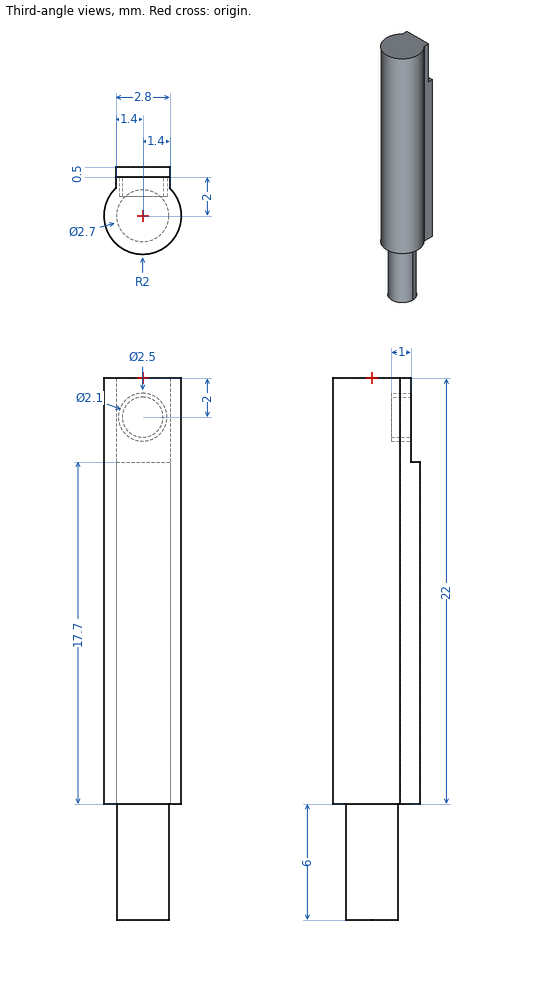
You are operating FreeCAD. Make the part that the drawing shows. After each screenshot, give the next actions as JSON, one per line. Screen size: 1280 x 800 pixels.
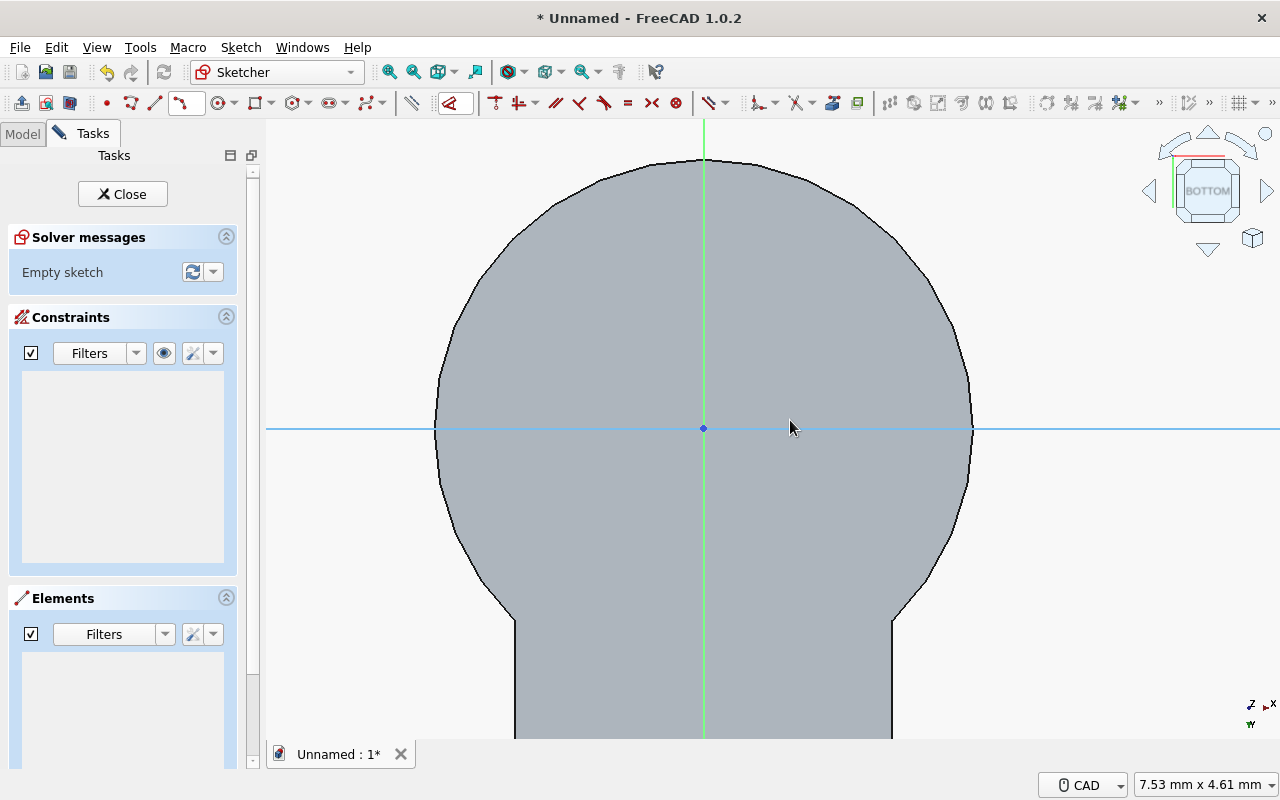
{"action": "left_click", "coordinate": [218, 104]}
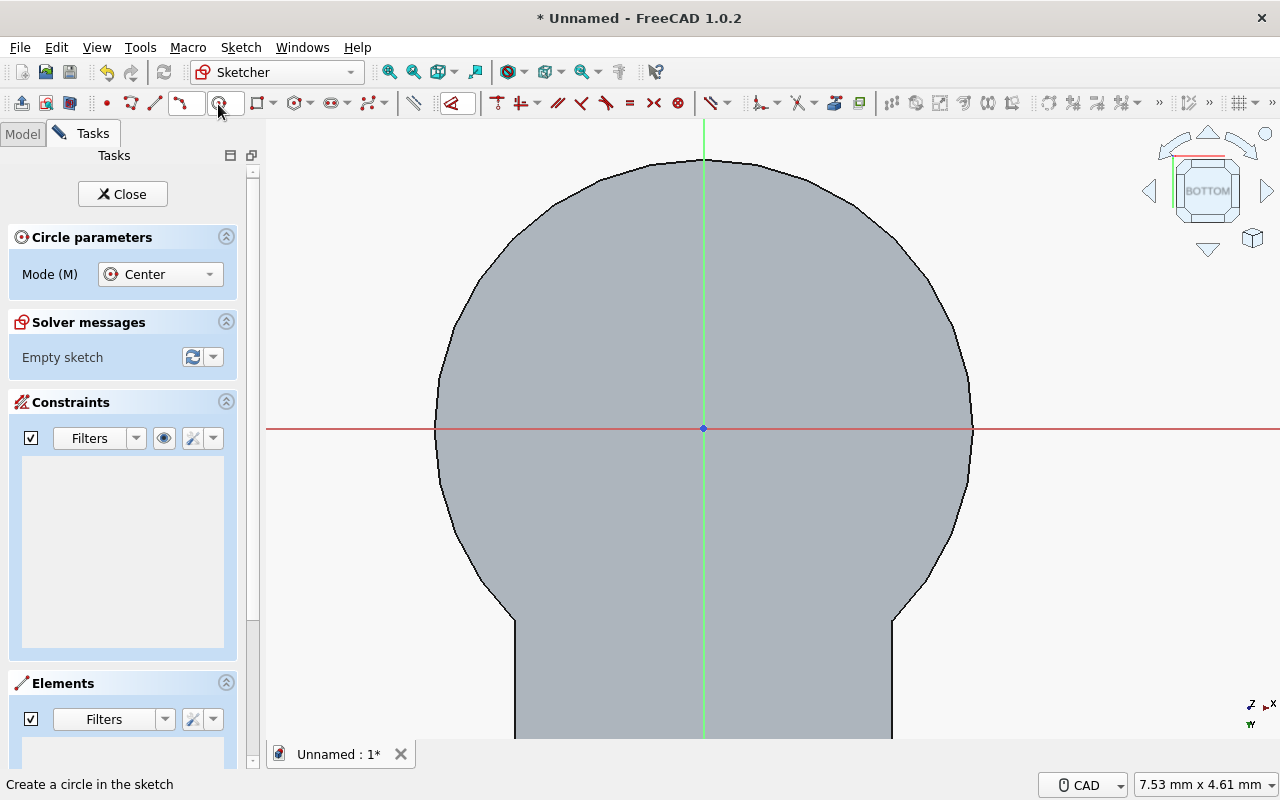
{"action": "left_click", "coordinate": [704, 429]}
{"action": "left_click", "coordinate": [832, 300]}
{"action": "key", "text": "Escape"}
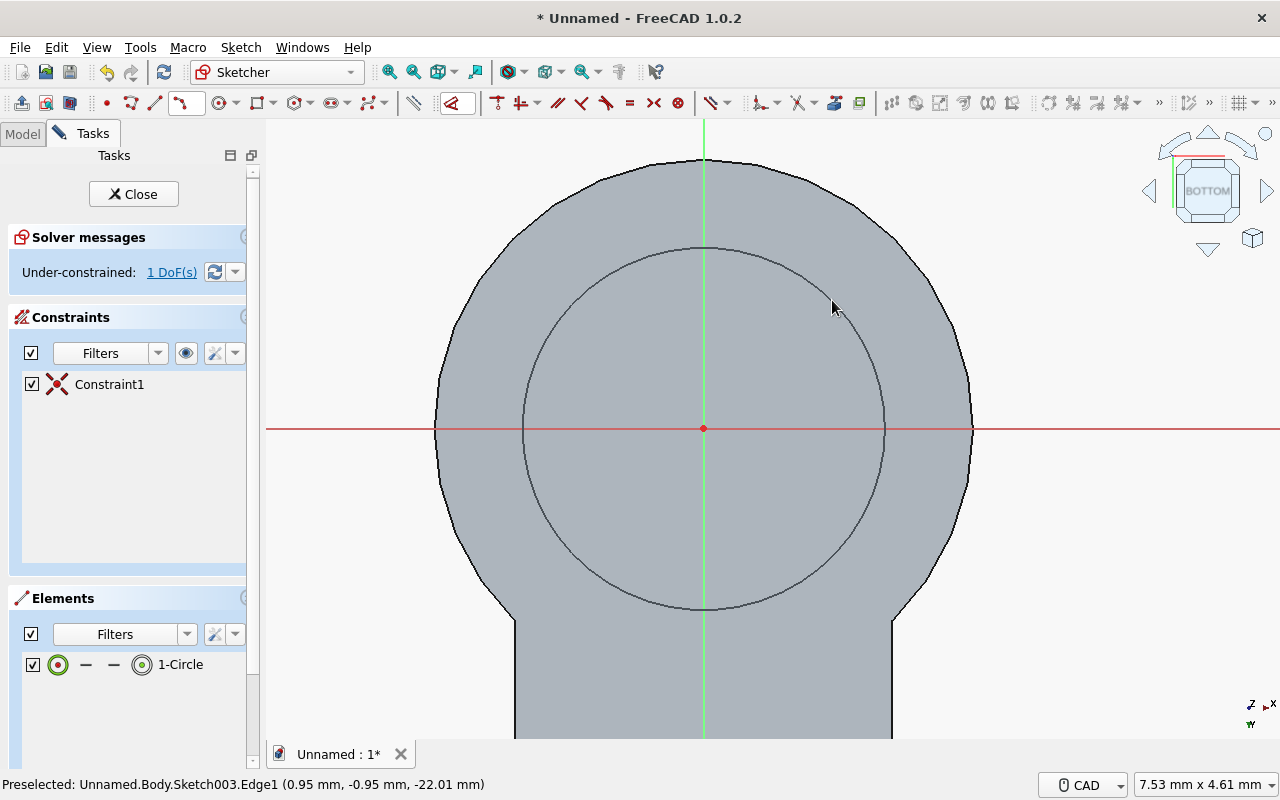
{"action": "left_click", "coordinate": [831, 300]}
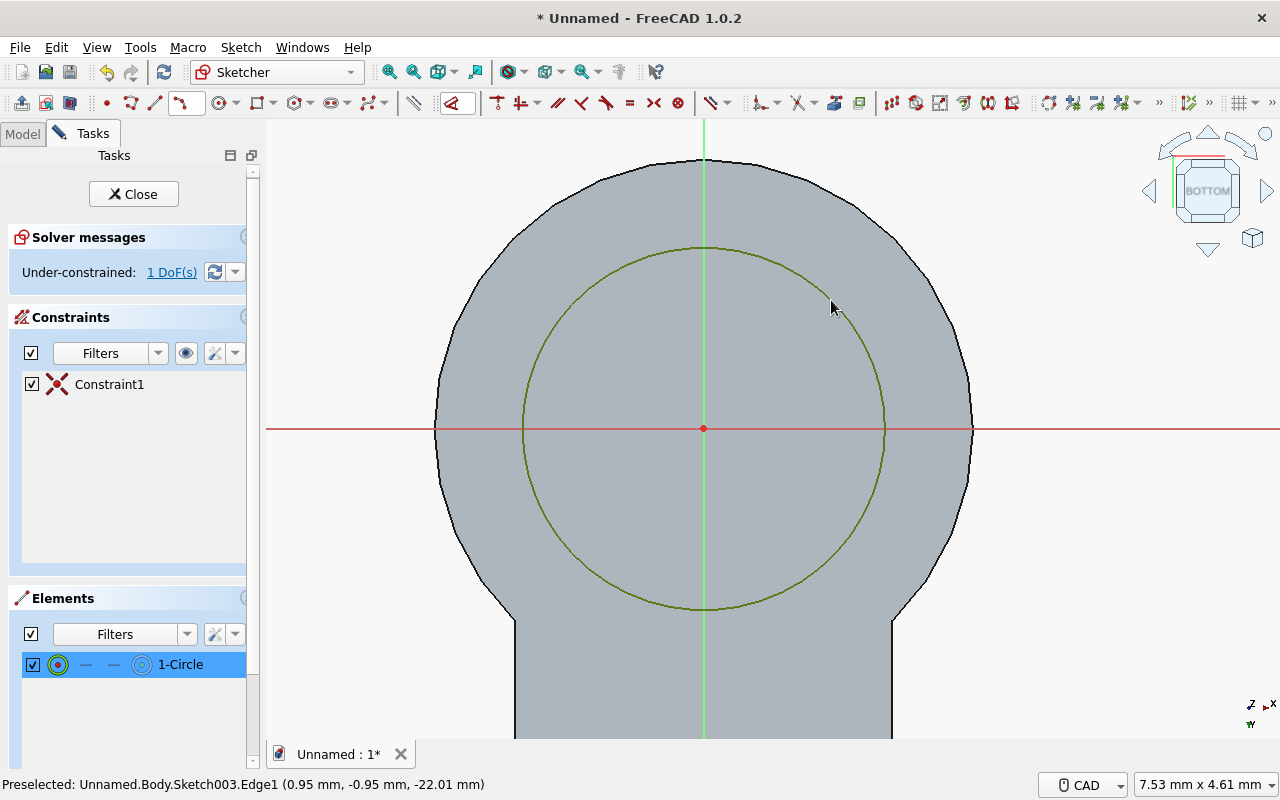
{"action": "left_click", "coordinate": [470, 104]}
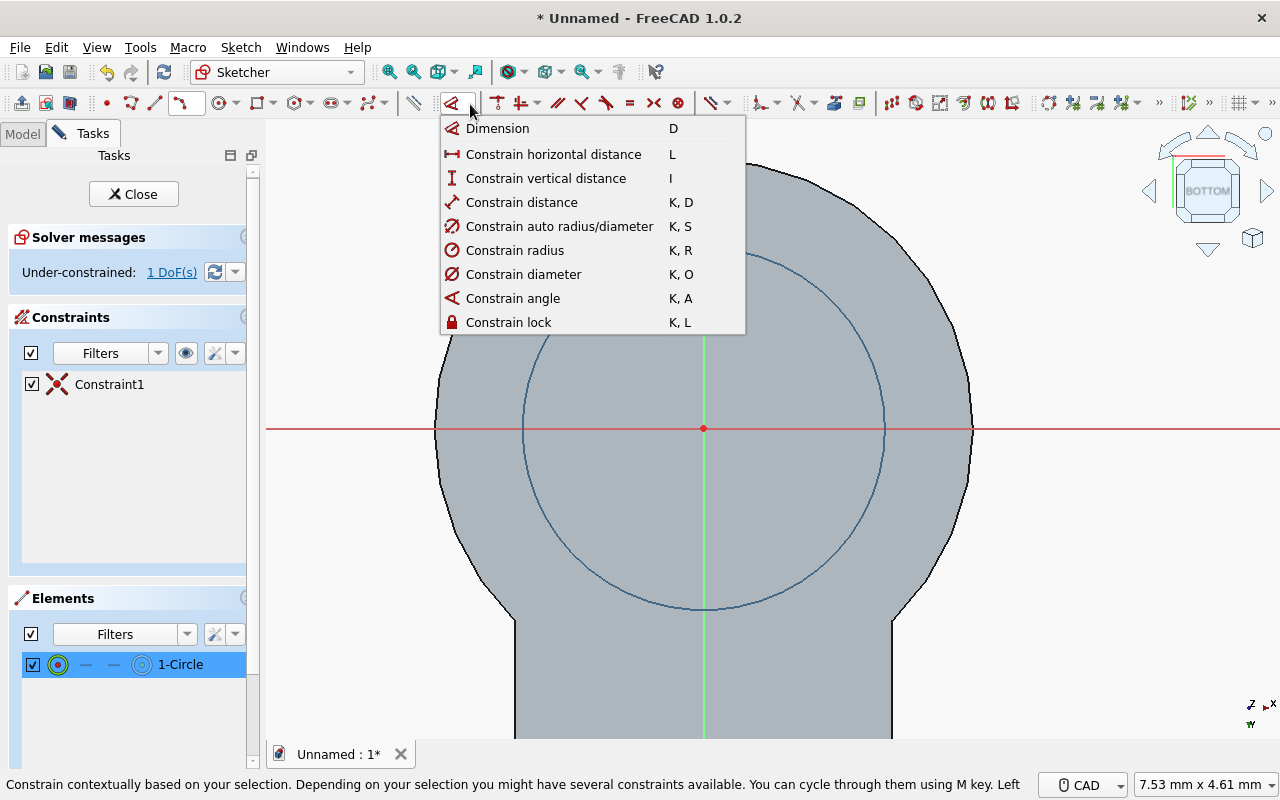
{"action": "left_click", "coordinate": [593, 274]}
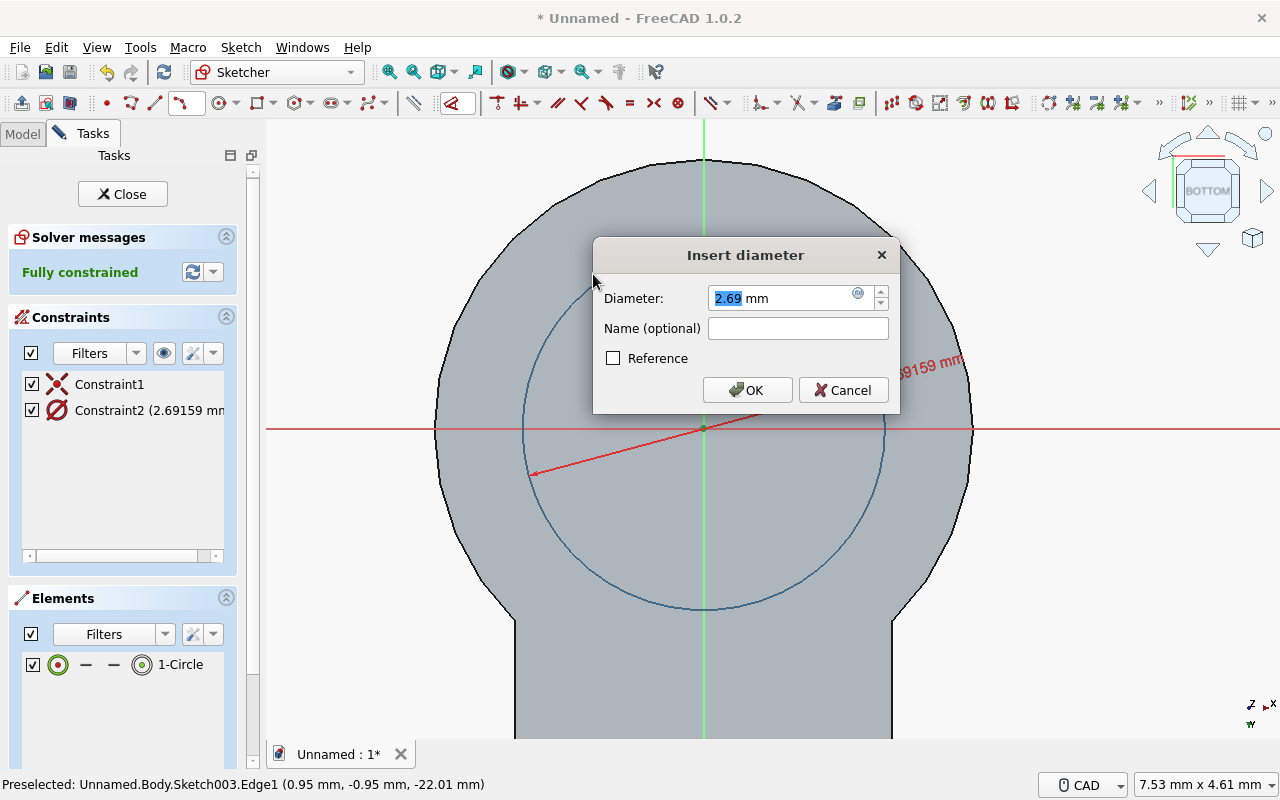
{"action": "type", "text": "2.7"}
{"action": "key", "text": "Return"}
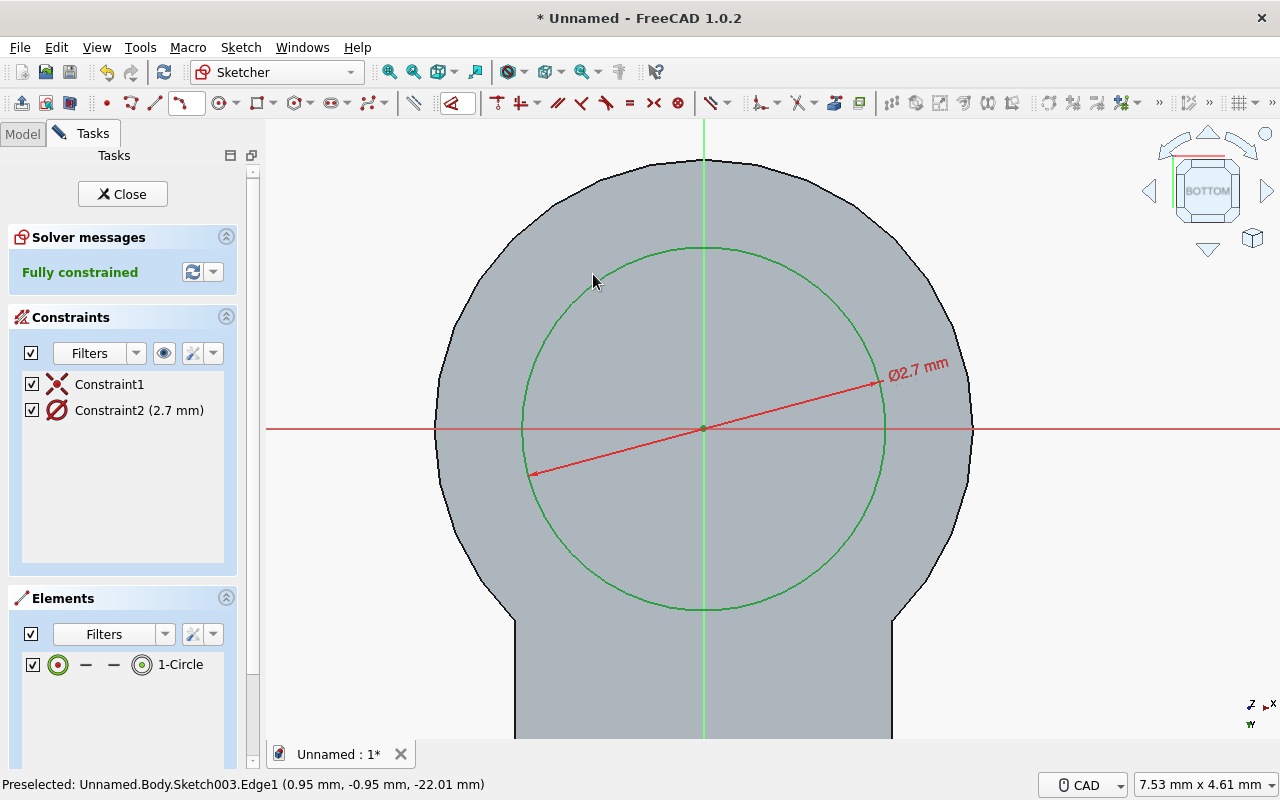
{"action": "left_click", "coordinate": [123, 194]}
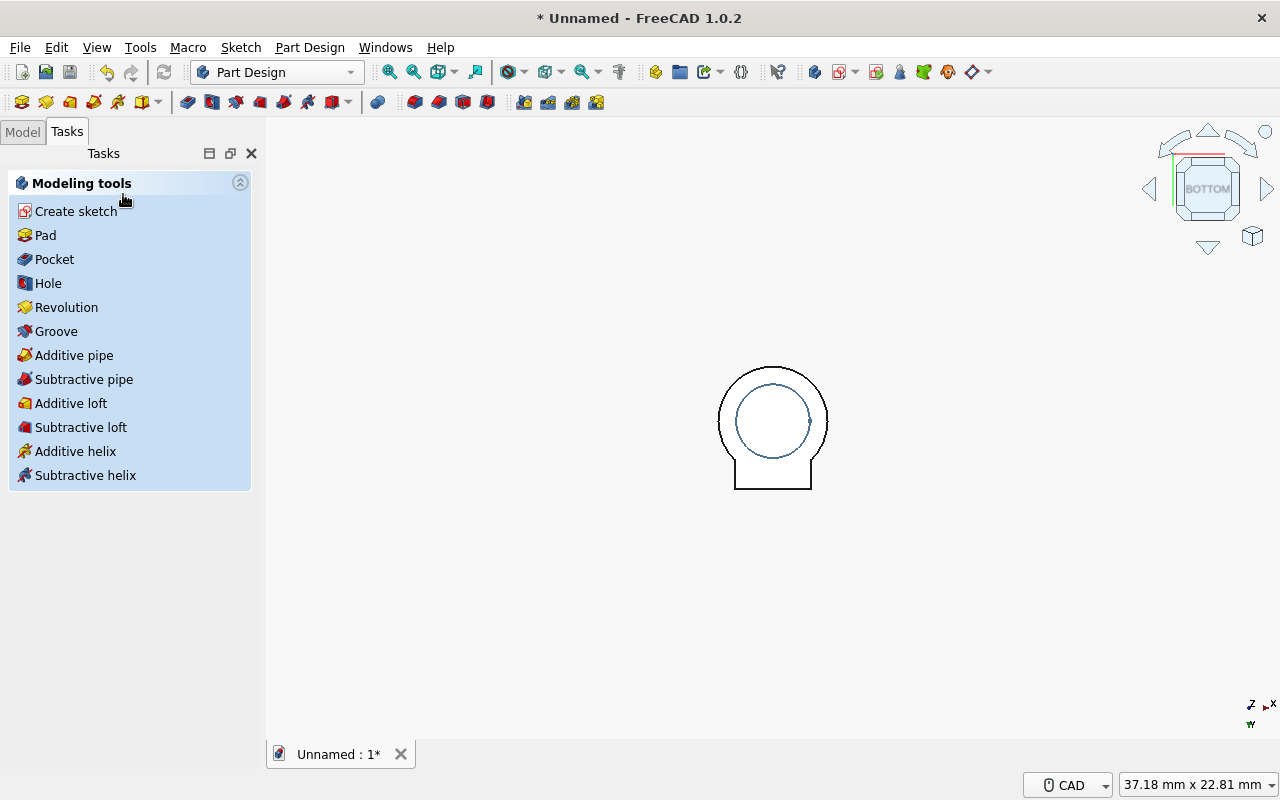
{"action": "left_click", "coordinate": [22, 102]}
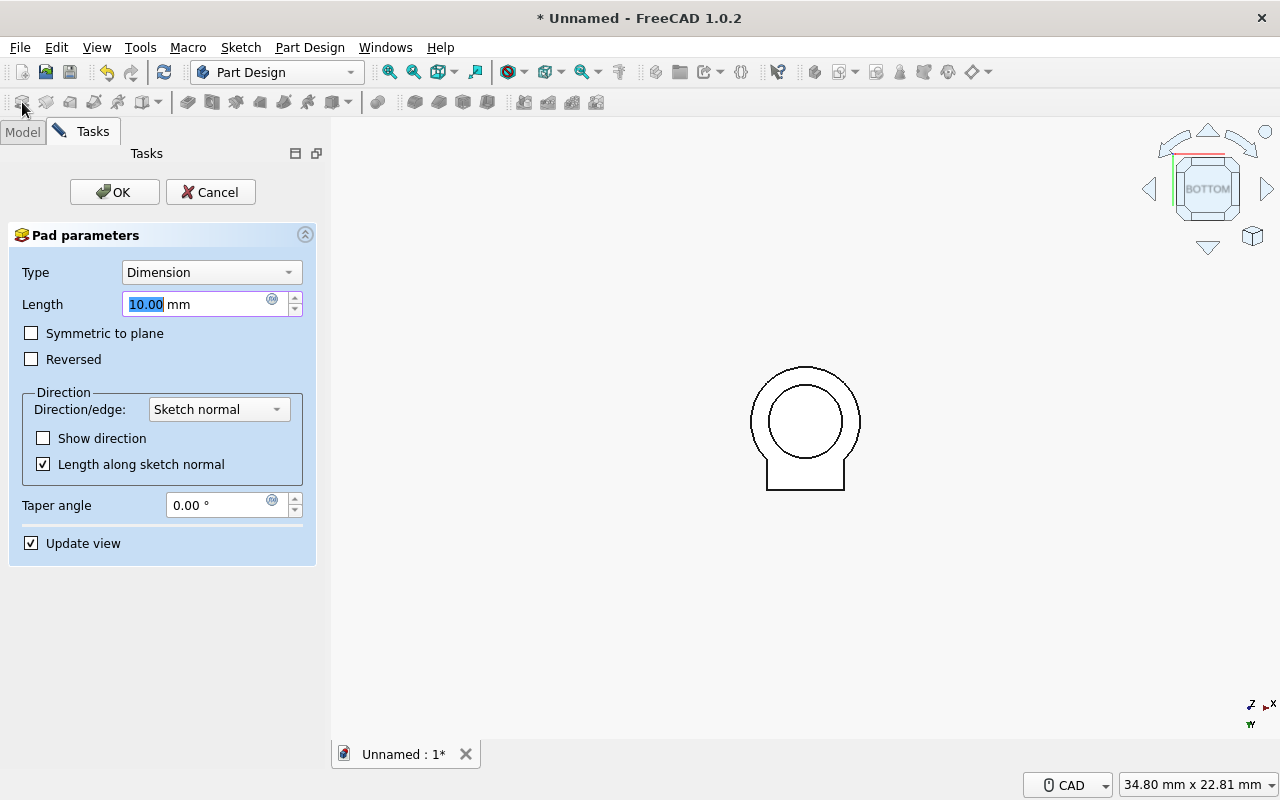
{"action": "type", "text": "6"}
{"action": "key", "text": "Tab"}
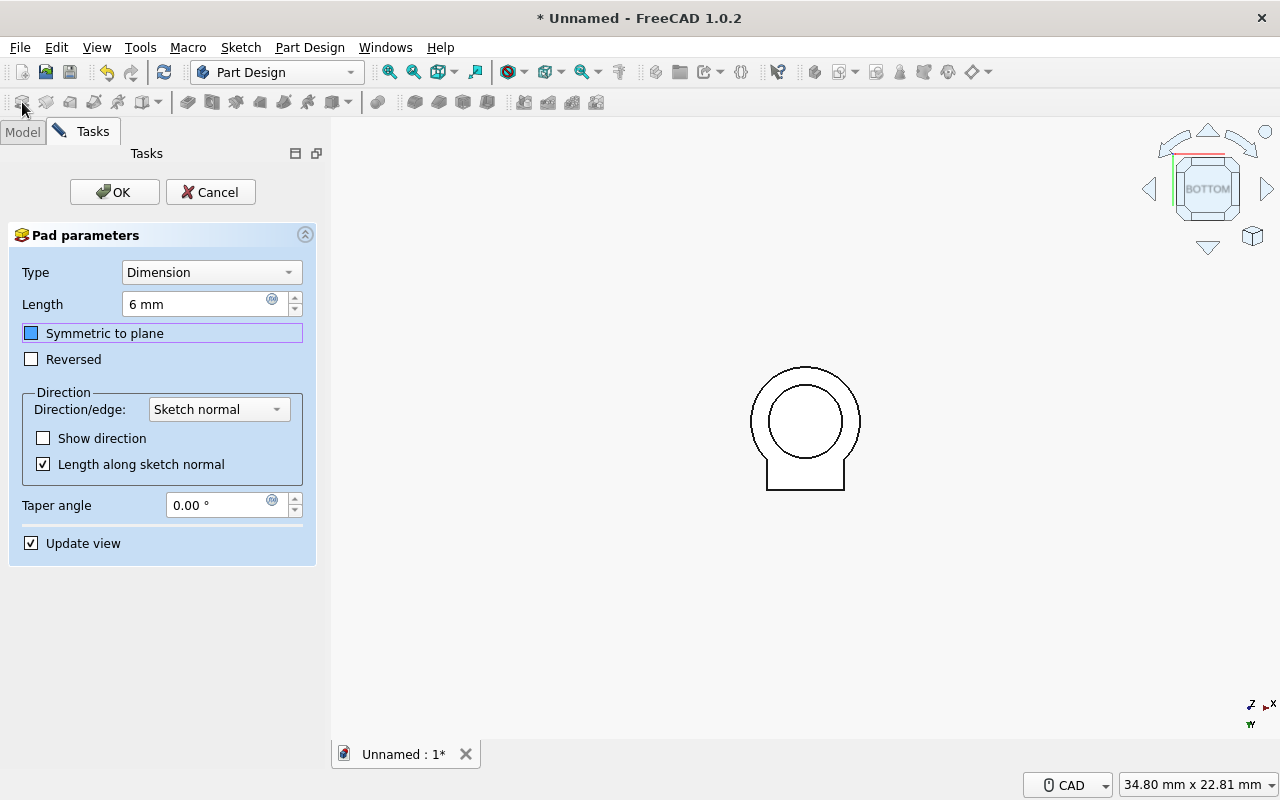
{"action": "left_click", "coordinate": [115, 192]}